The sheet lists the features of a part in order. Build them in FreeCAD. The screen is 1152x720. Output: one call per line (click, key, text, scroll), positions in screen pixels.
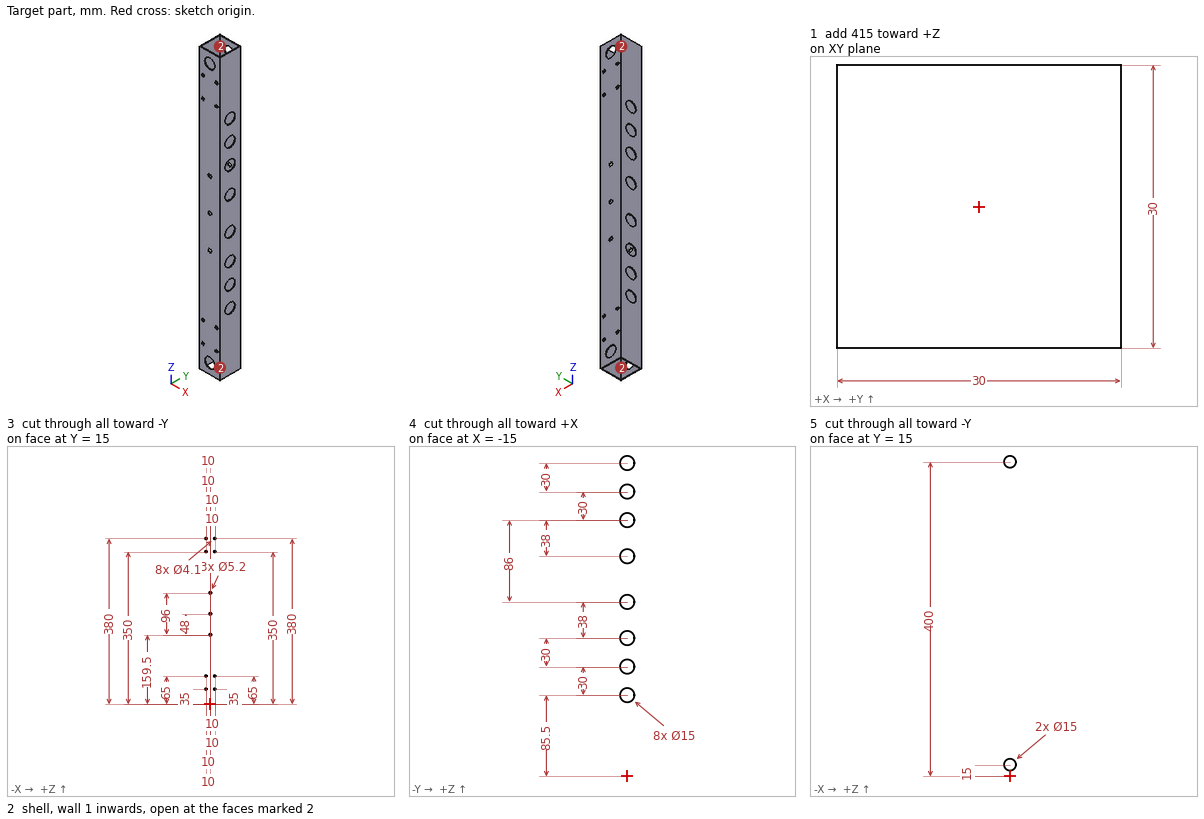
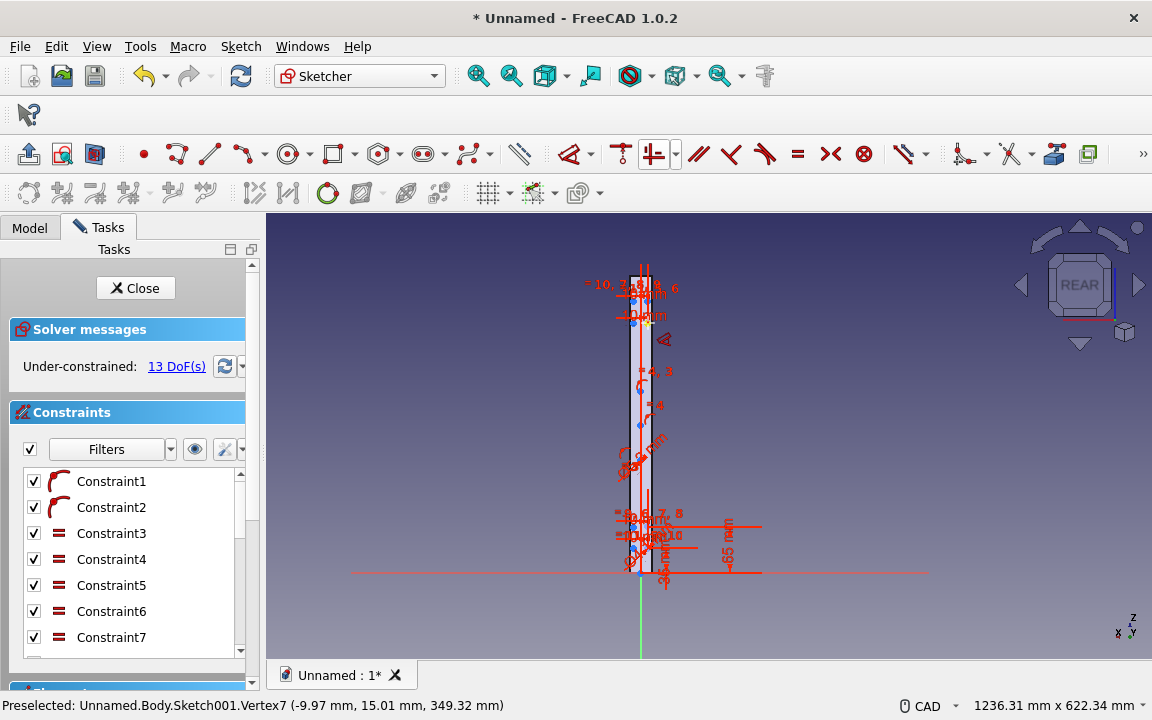
scroll(634, 527, up, 9)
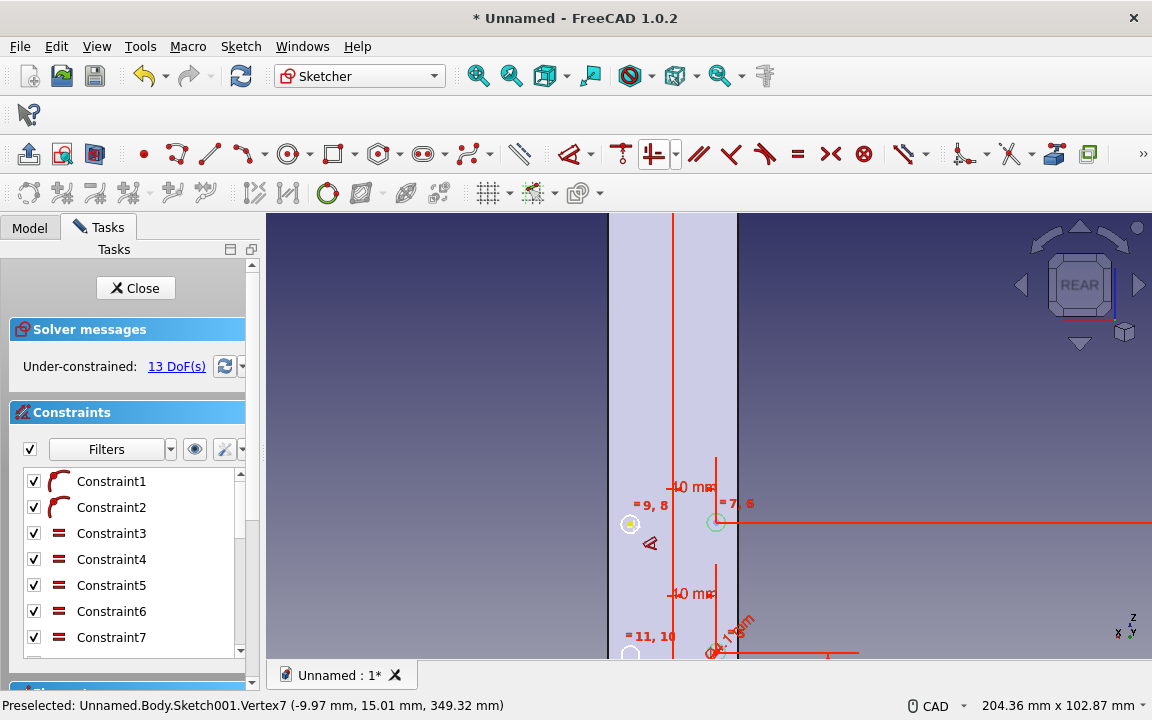
click(630, 524)
click(652, 466)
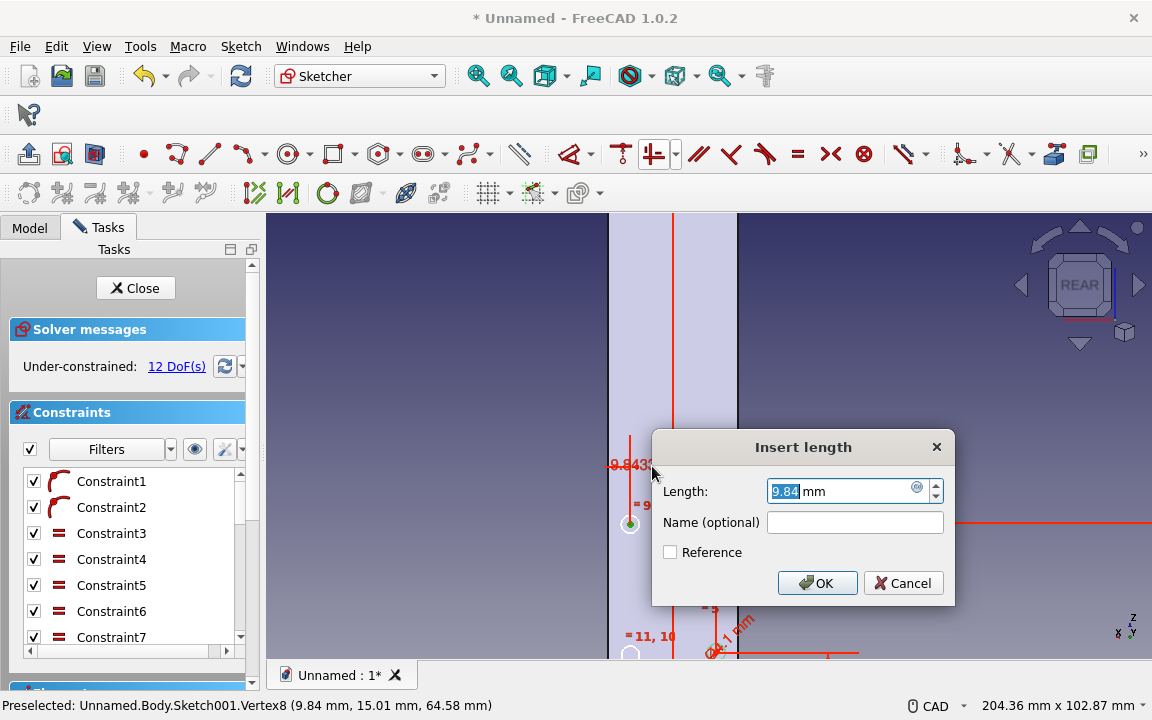
text(10)
key(Return)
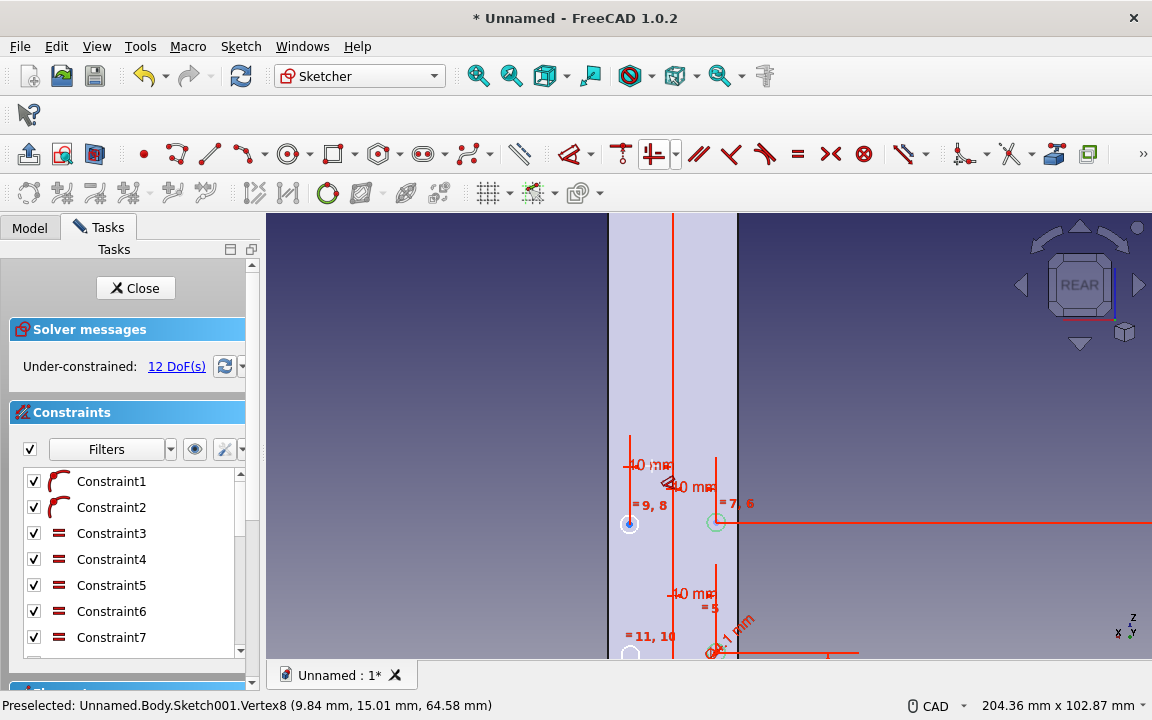
scroll(634, 527, down, 9)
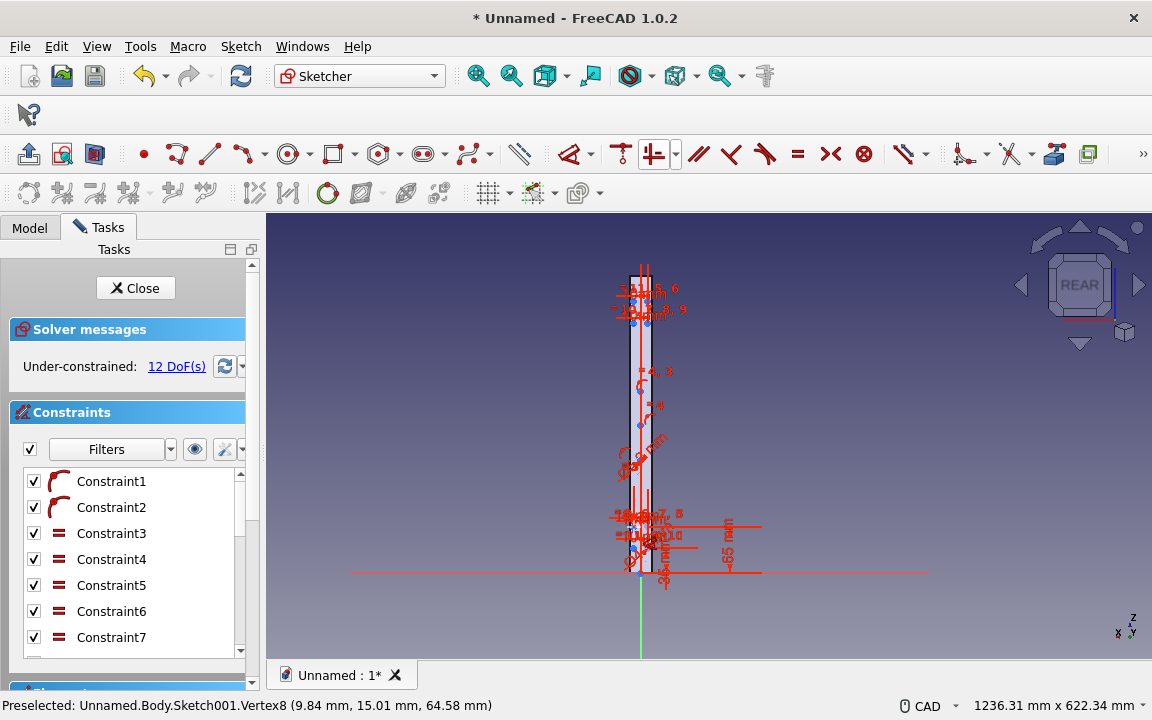
click(634, 527)
click(552, 550)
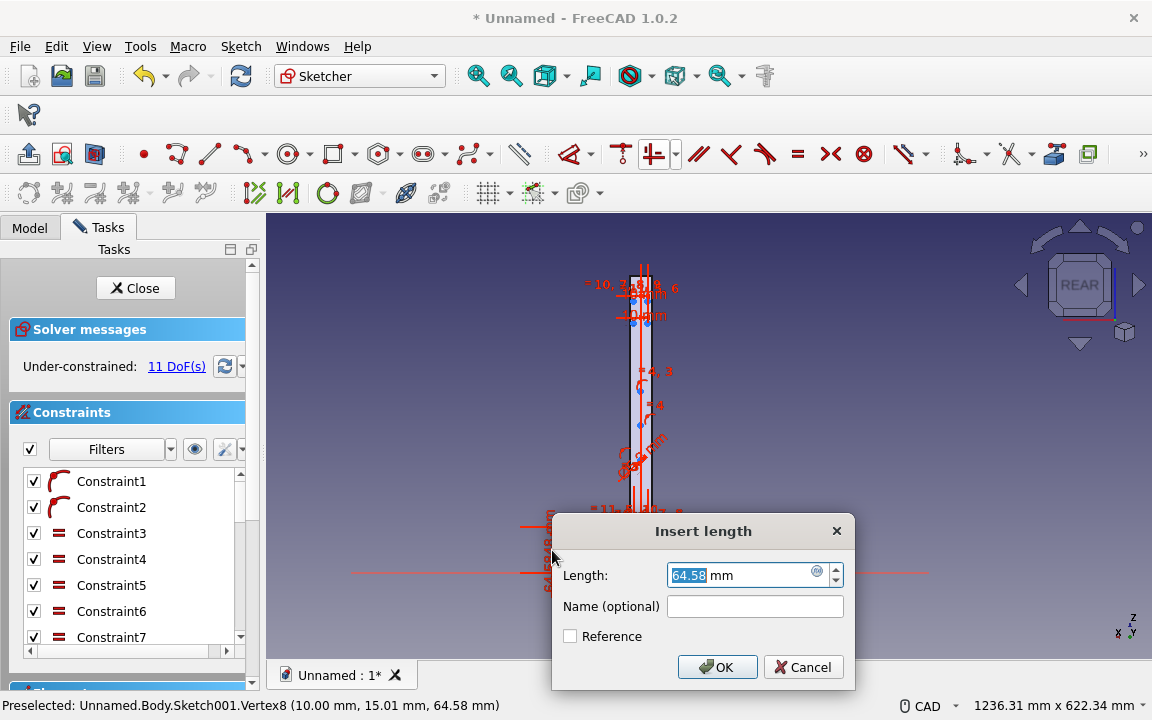
text(65)
key(Return)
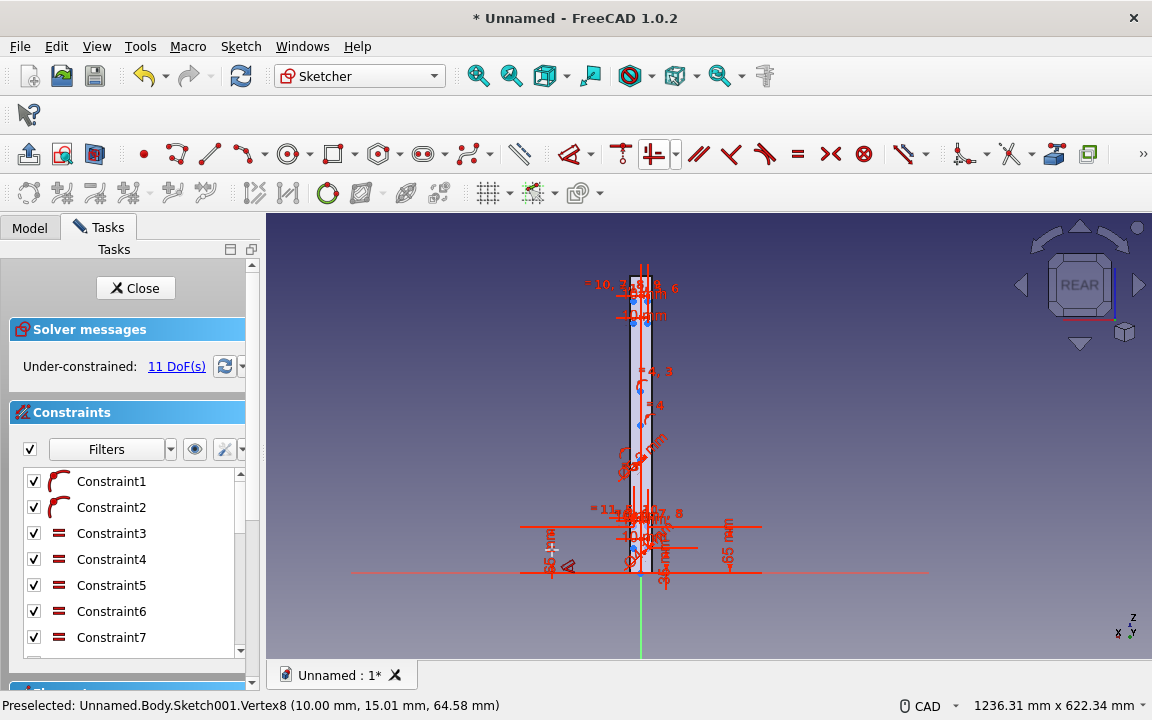
scroll(633, 323, up, 9)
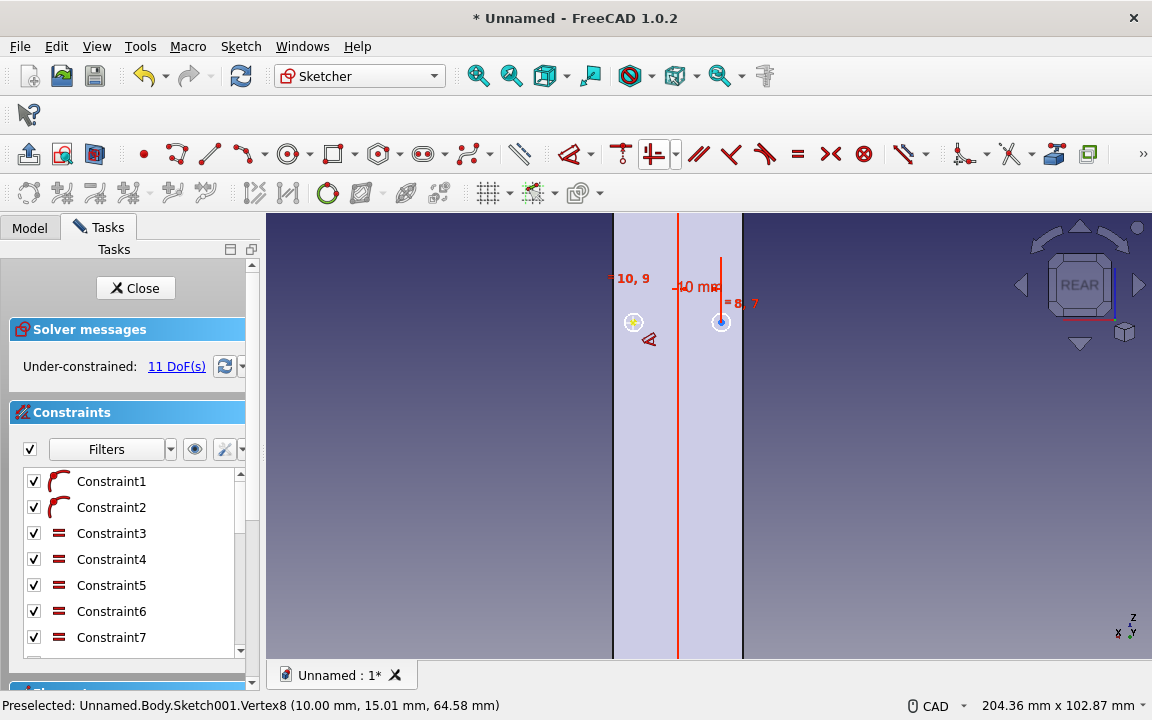
click(634, 322)
click(656, 264)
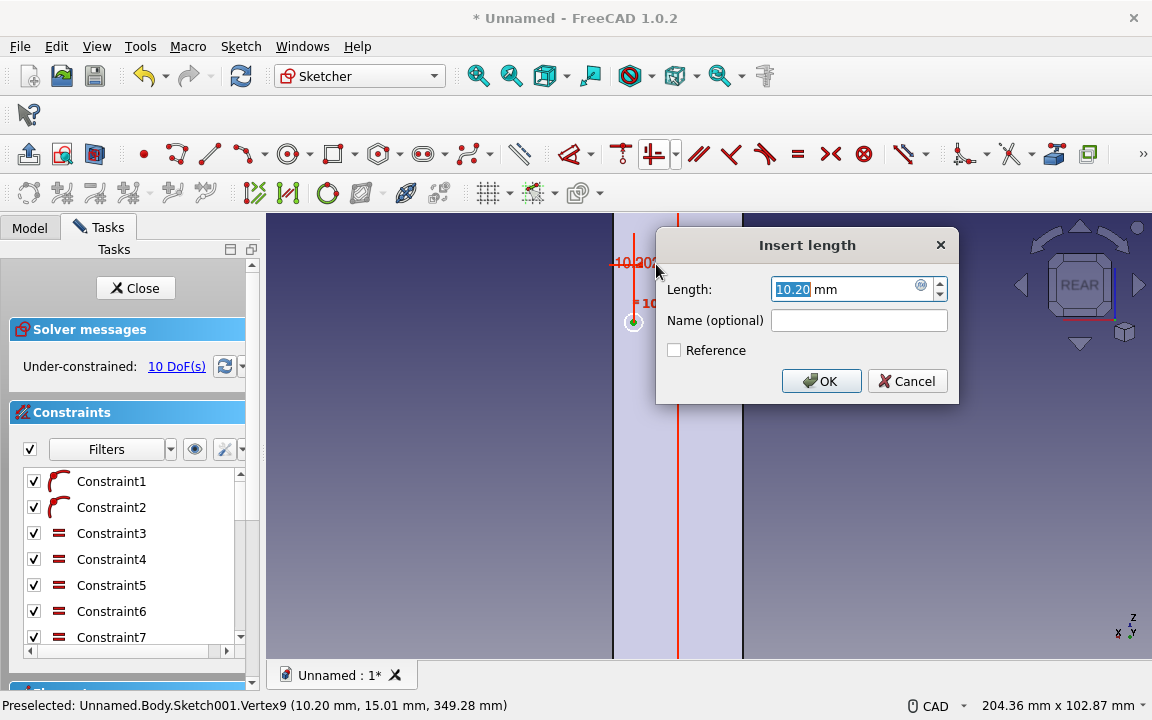
text(10)
key(Return)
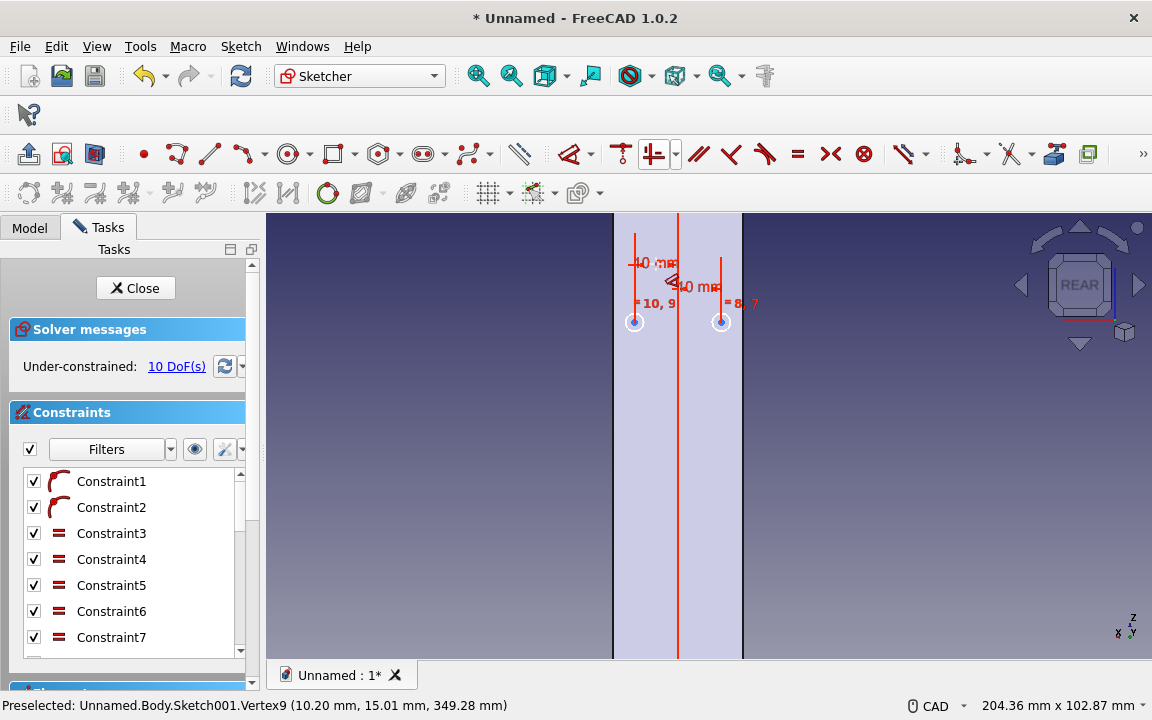
scroll(633, 323, down, 9)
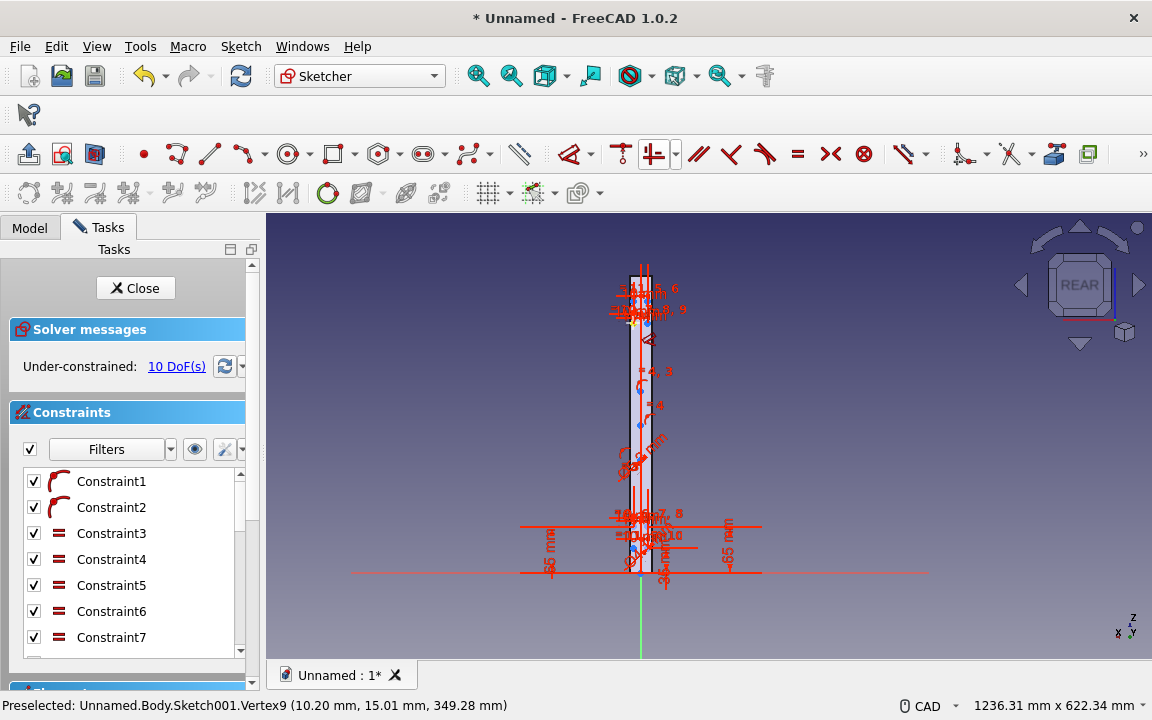
scroll(634, 549, up, 9)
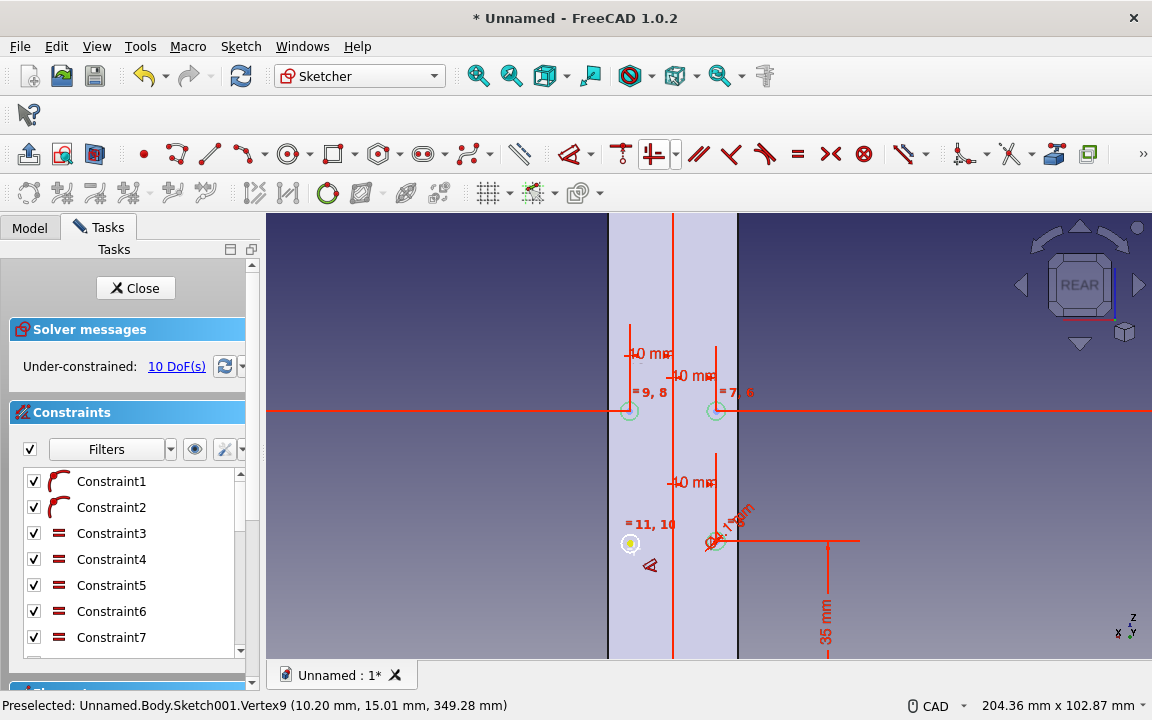
click(630, 544)
click(652, 510)